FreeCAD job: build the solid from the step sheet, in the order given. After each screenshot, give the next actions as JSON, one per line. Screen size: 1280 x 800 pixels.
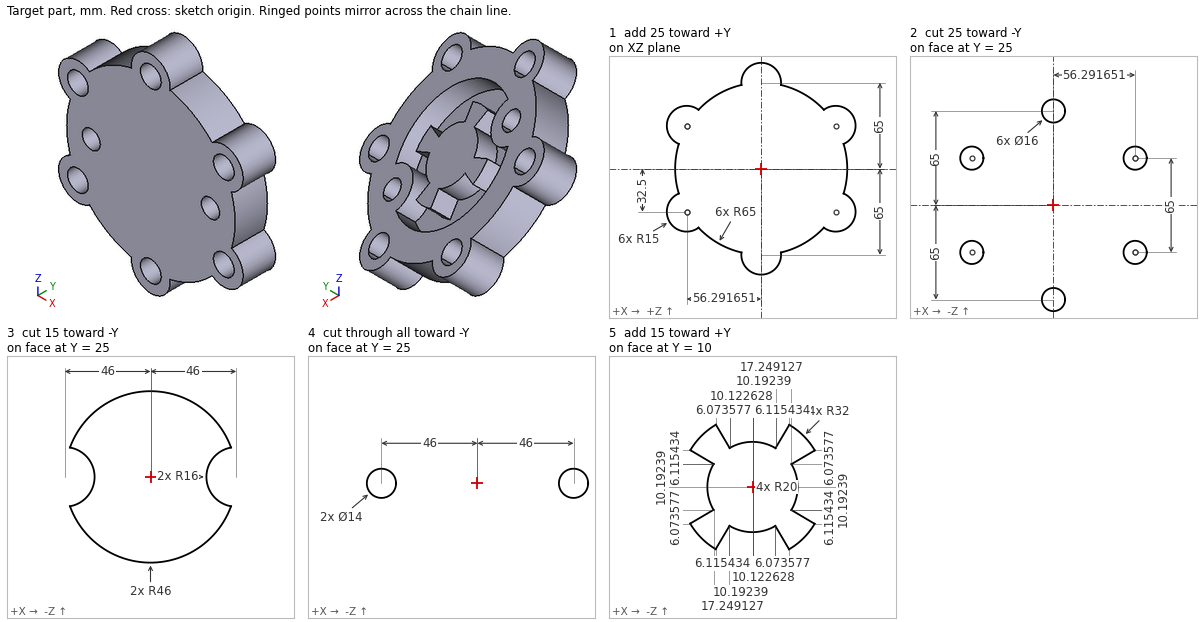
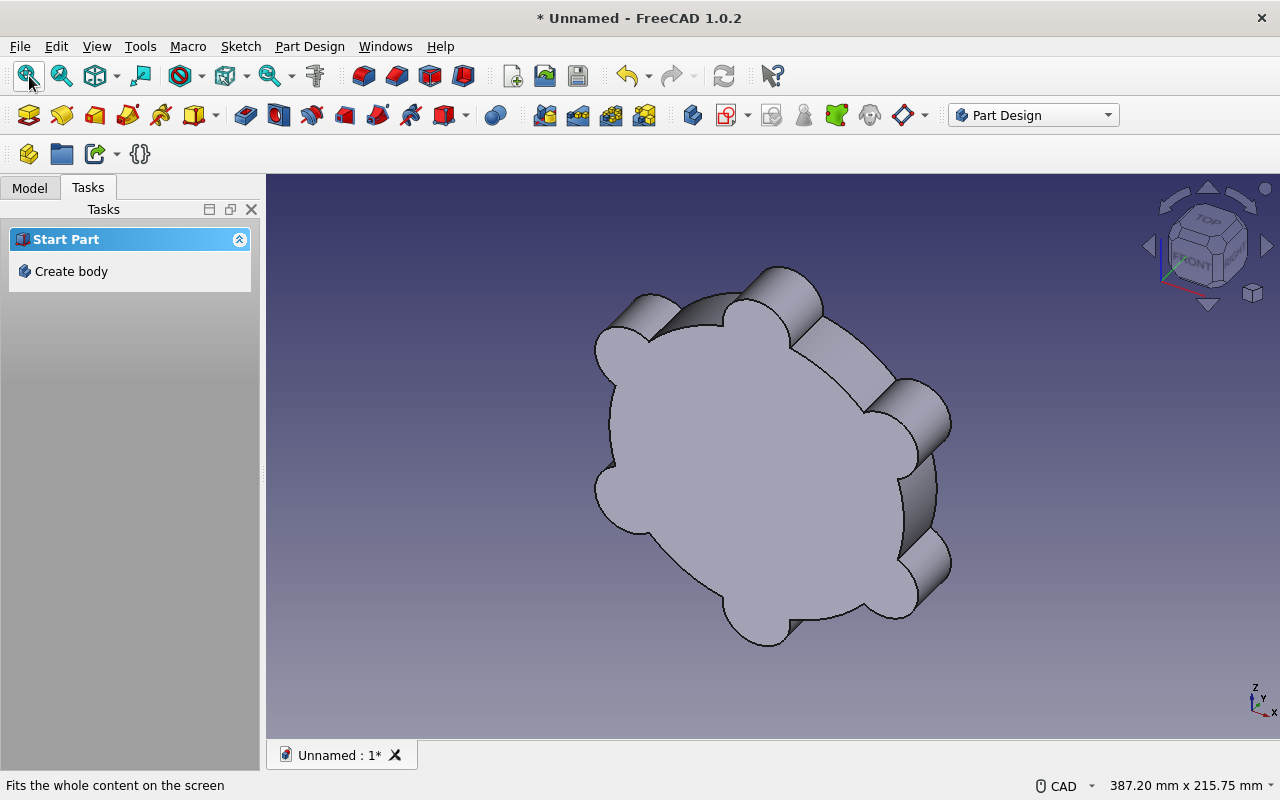
{"action": "key", "text": "4"}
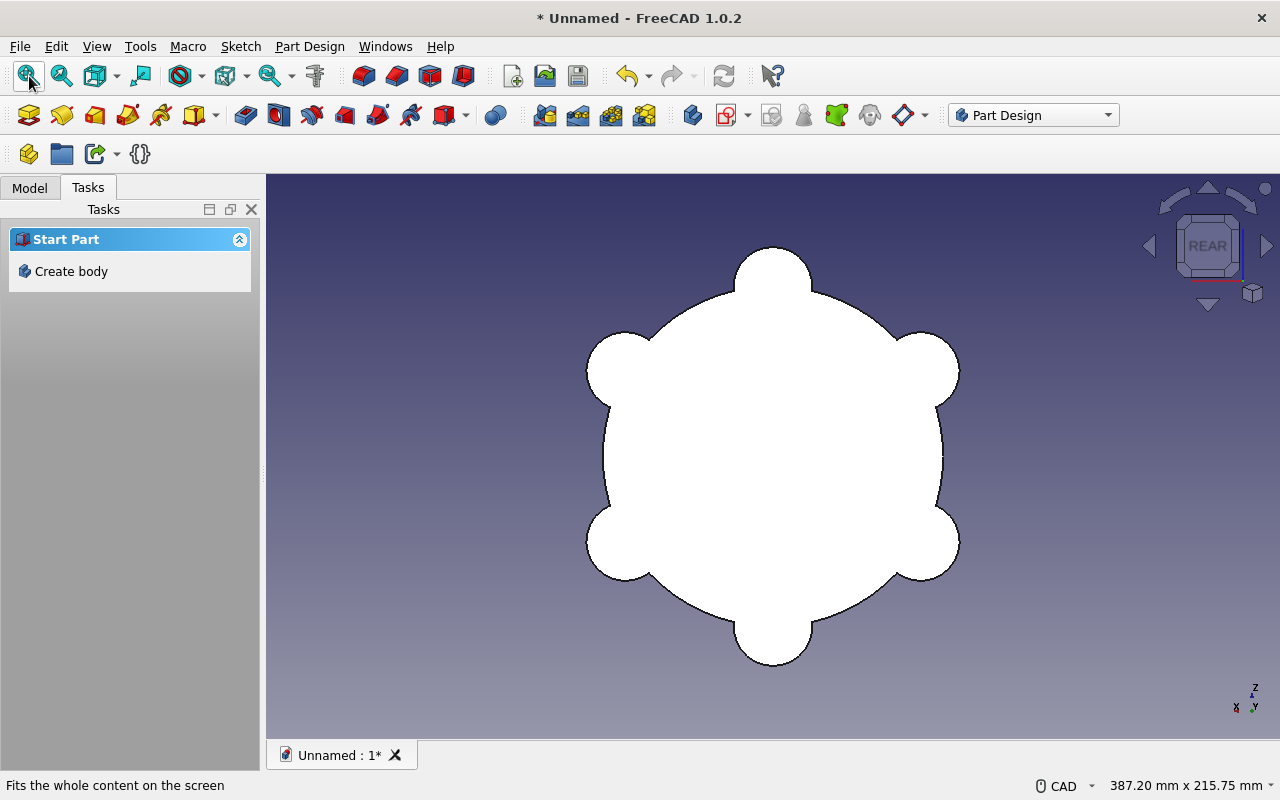
{"action": "left_click", "coordinate": [773, 455]}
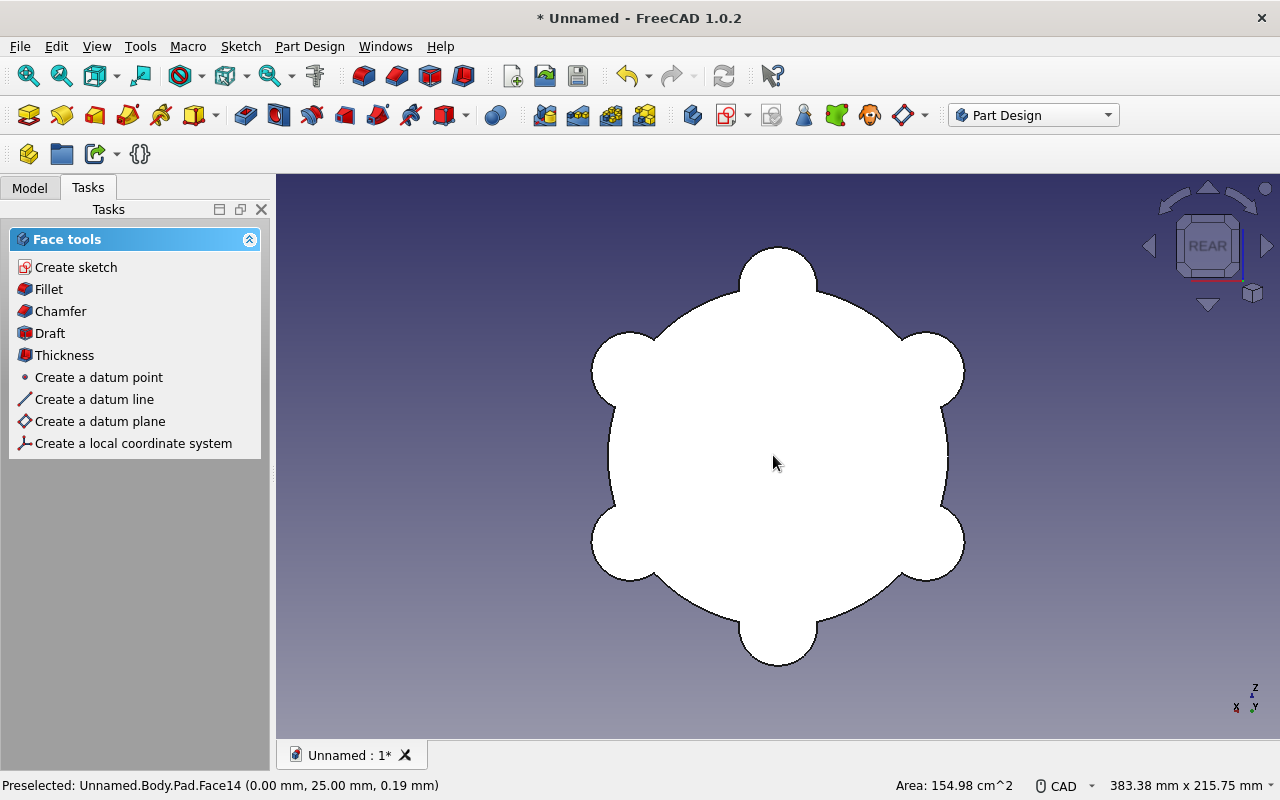
{"action": "left_click", "coordinate": [726, 116]}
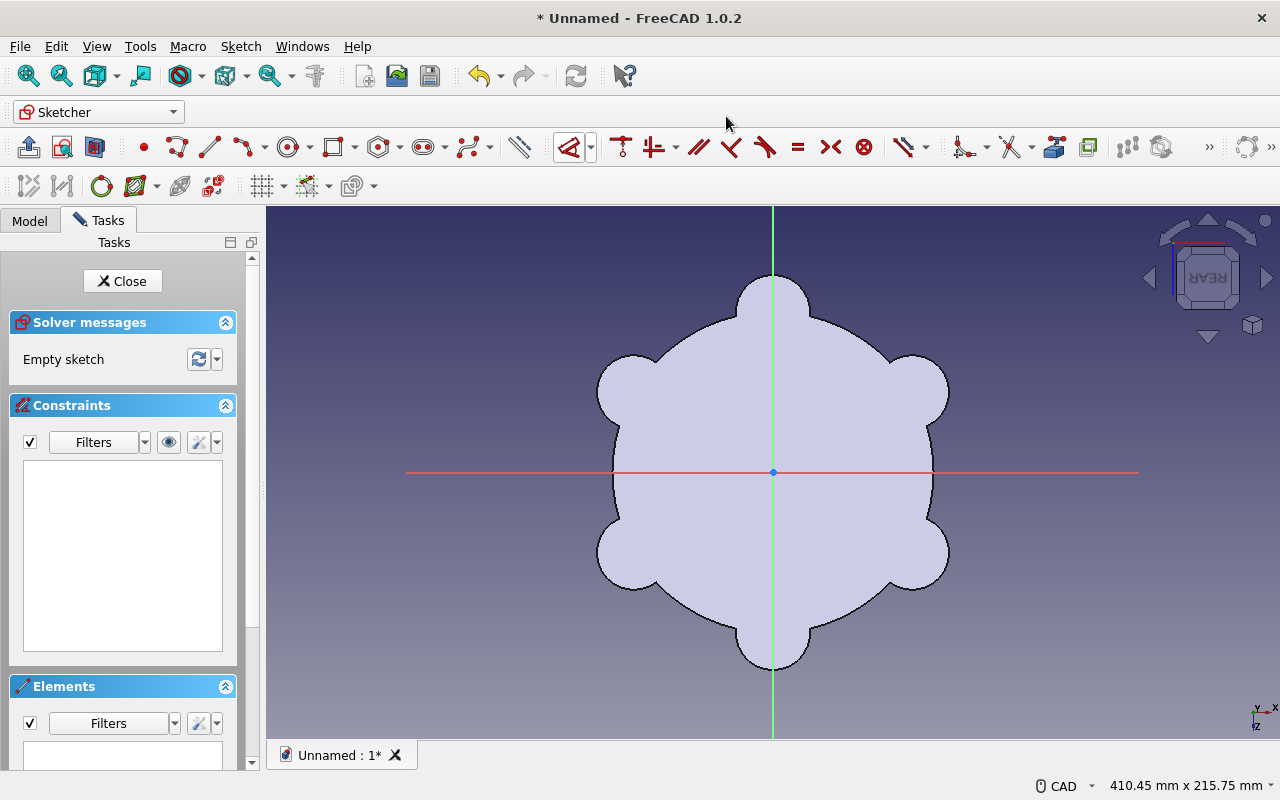
{"action": "left_click", "coordinate": [288, 148]}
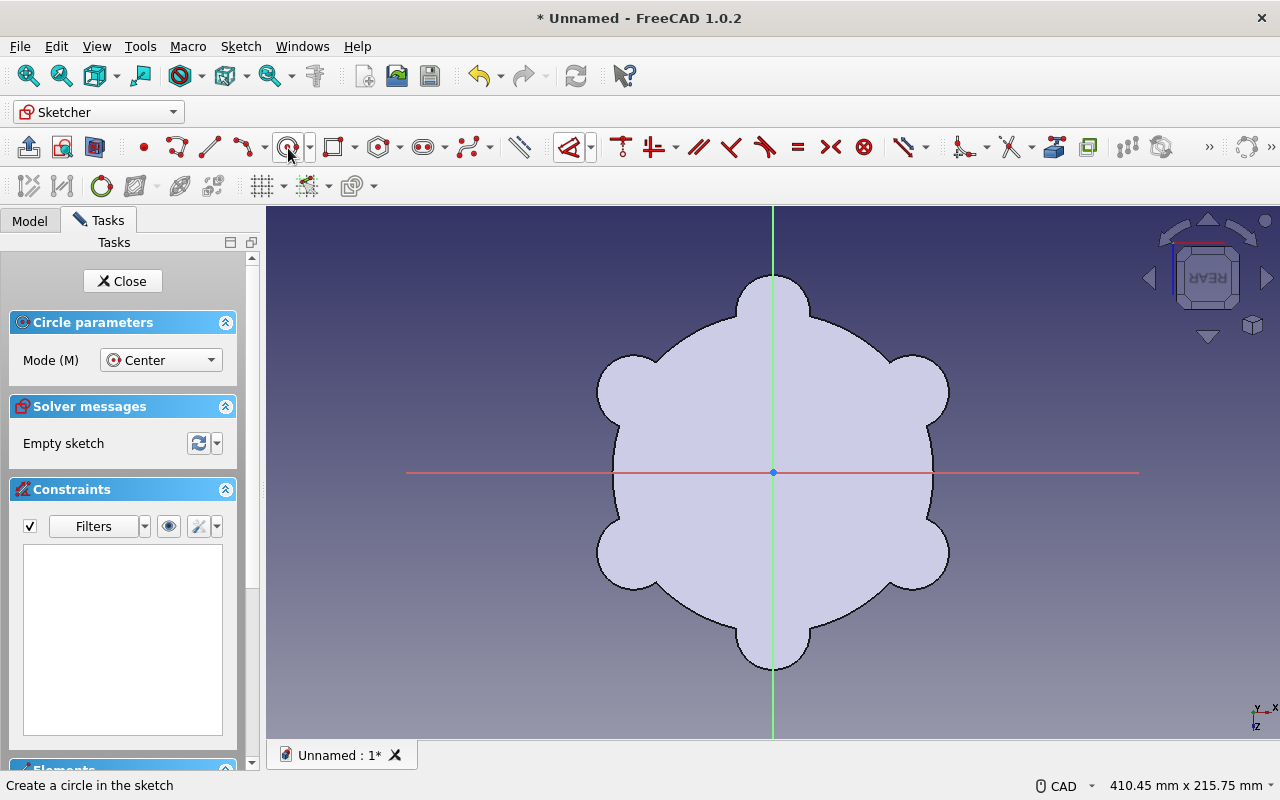
{"action": "left_click", "coordinate": [773, 312]}
{"action": "mouse_move", "coordinate": [792, 305]}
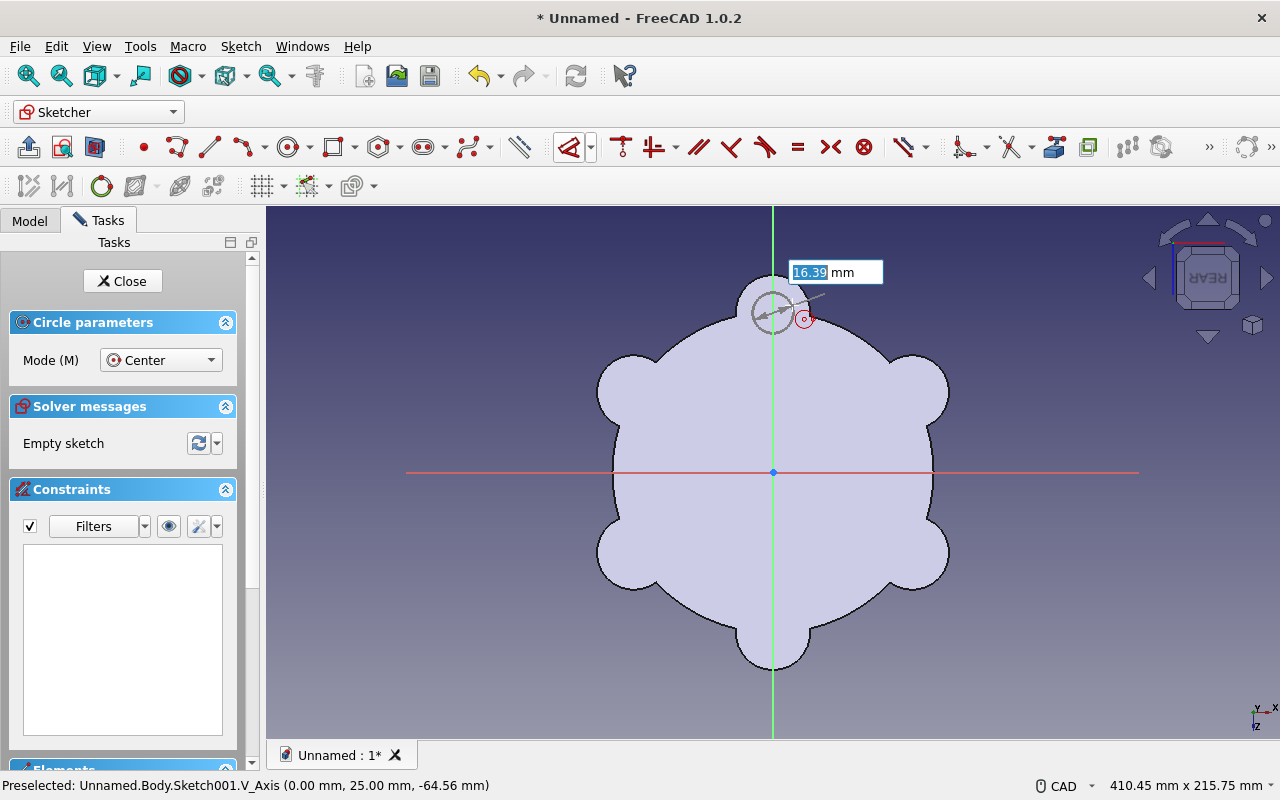
{"action": "type", "text": "16"}
{"action": "key", "text": "Return"}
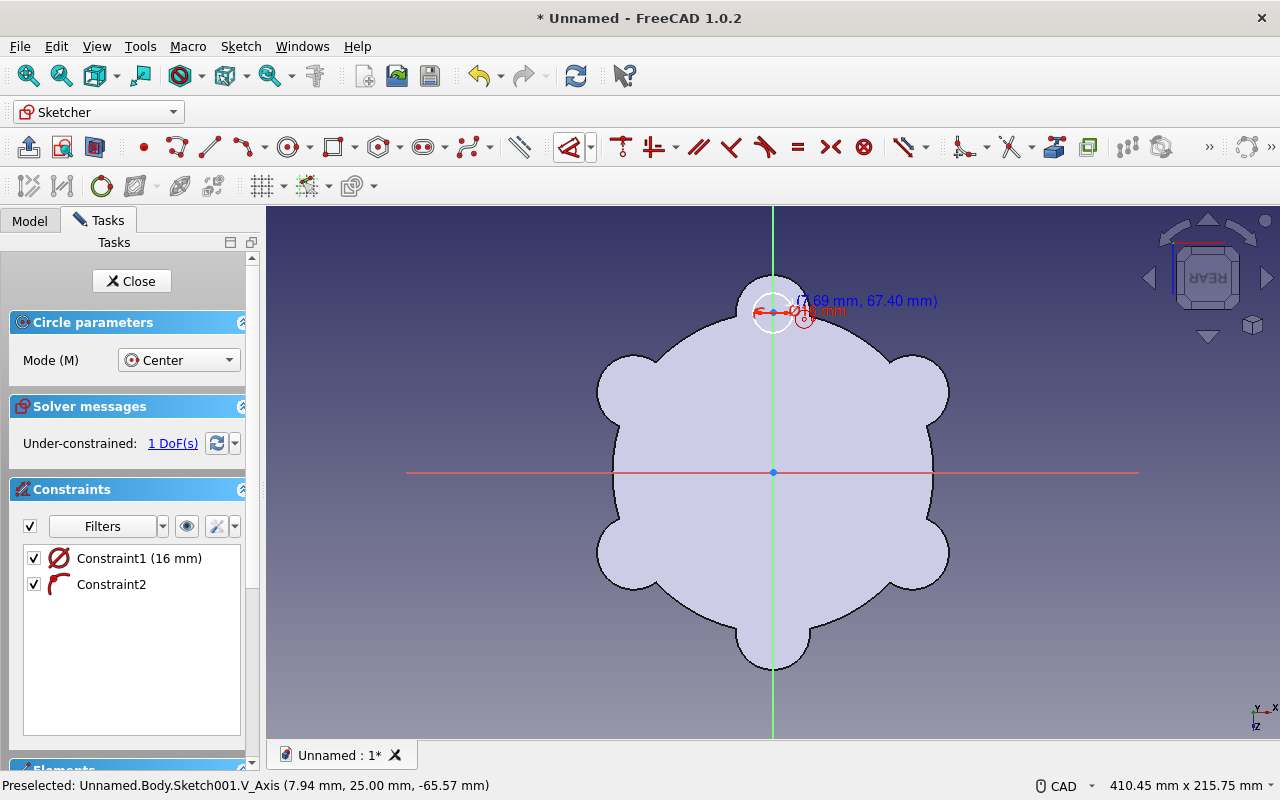
{"action": "left_click", "coordinate": [912, 392]}
{"action": "mouse_move", "coordinate": [926, 378]}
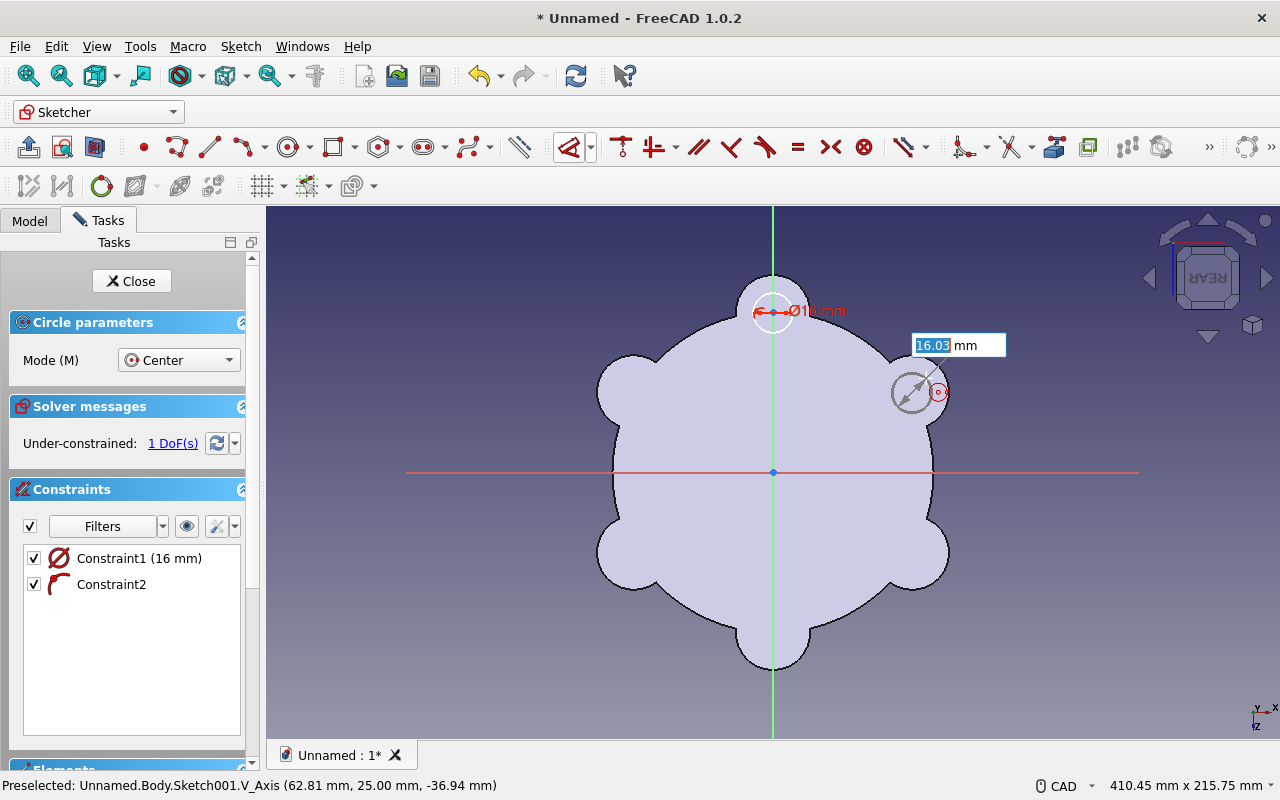
{"action": "type", "text": "16"}
{"action": "key", "text": "Return"}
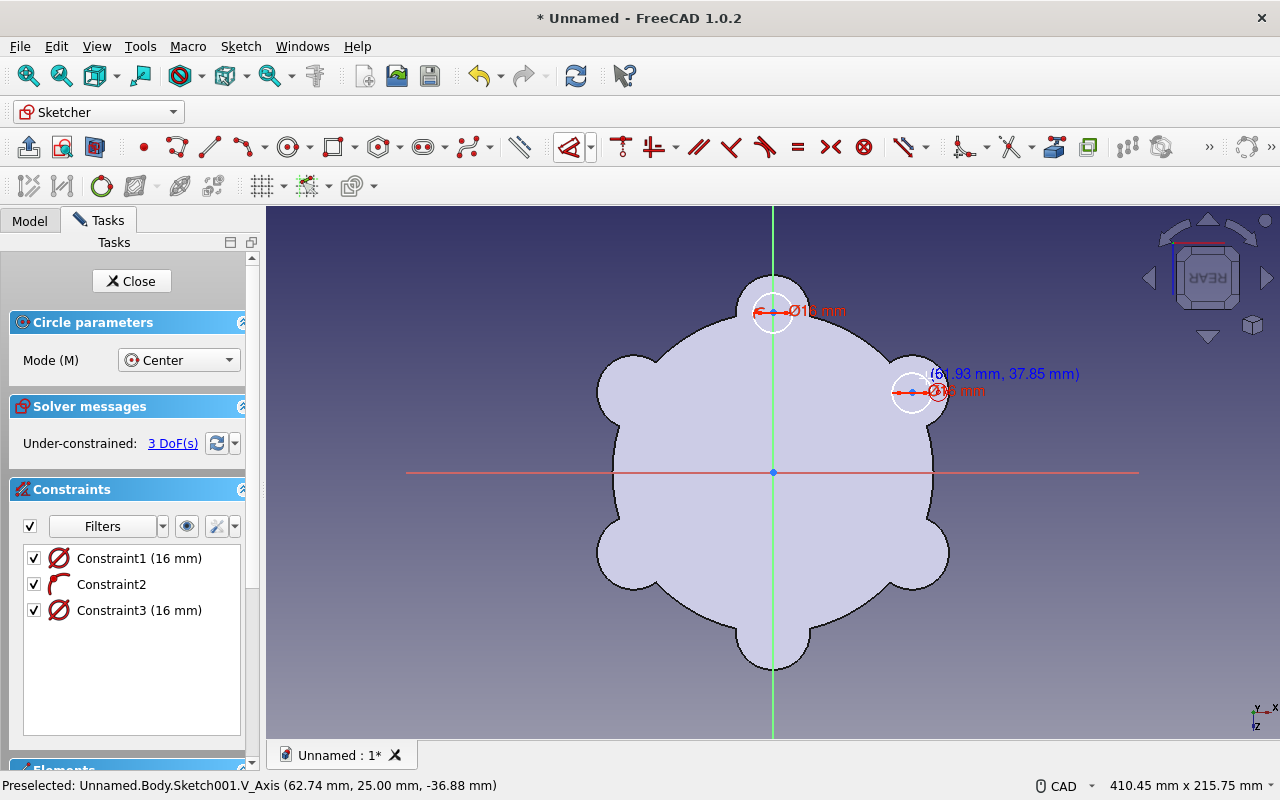
{"action": "left_click", "coordinate": [912, 553]}
{"action": "mouse_move", "coordinate": [926, 539]}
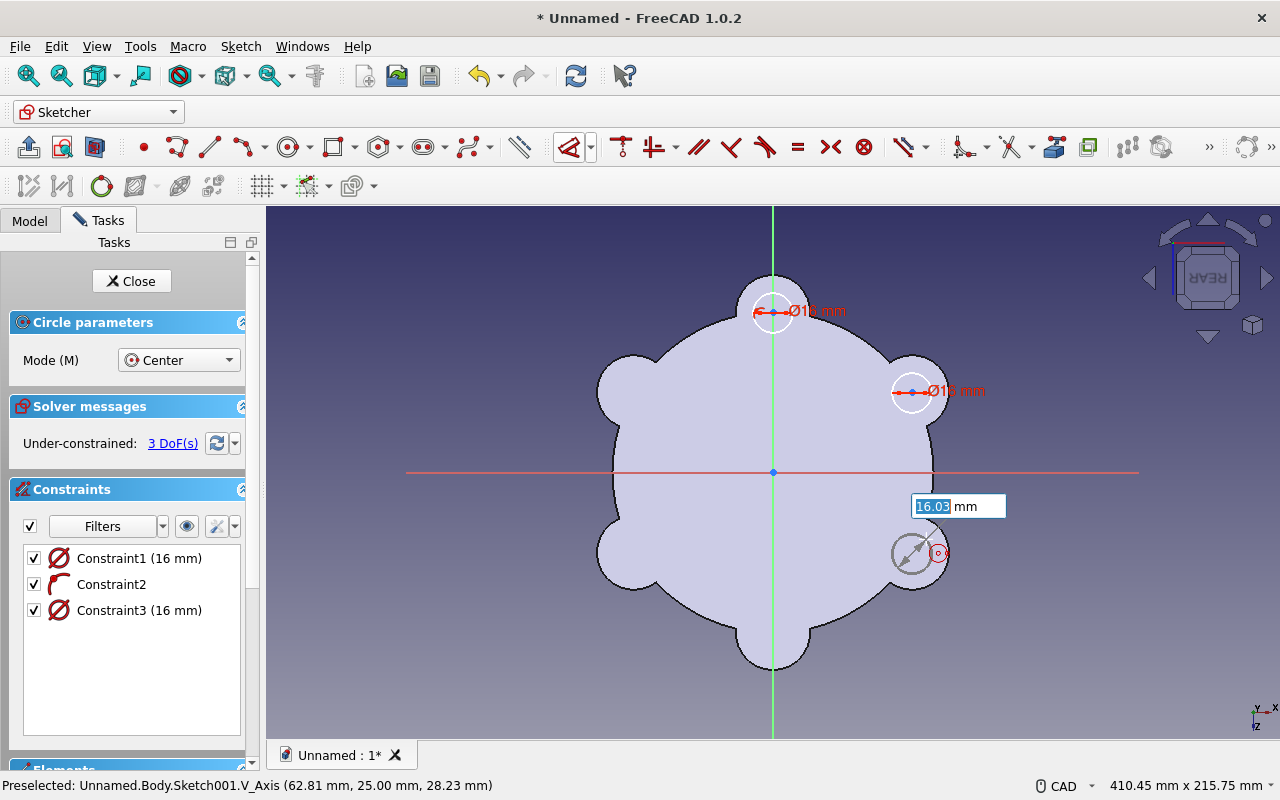
{"action": "type", "text": "16"}
{"action": "key", "text": "Return"}